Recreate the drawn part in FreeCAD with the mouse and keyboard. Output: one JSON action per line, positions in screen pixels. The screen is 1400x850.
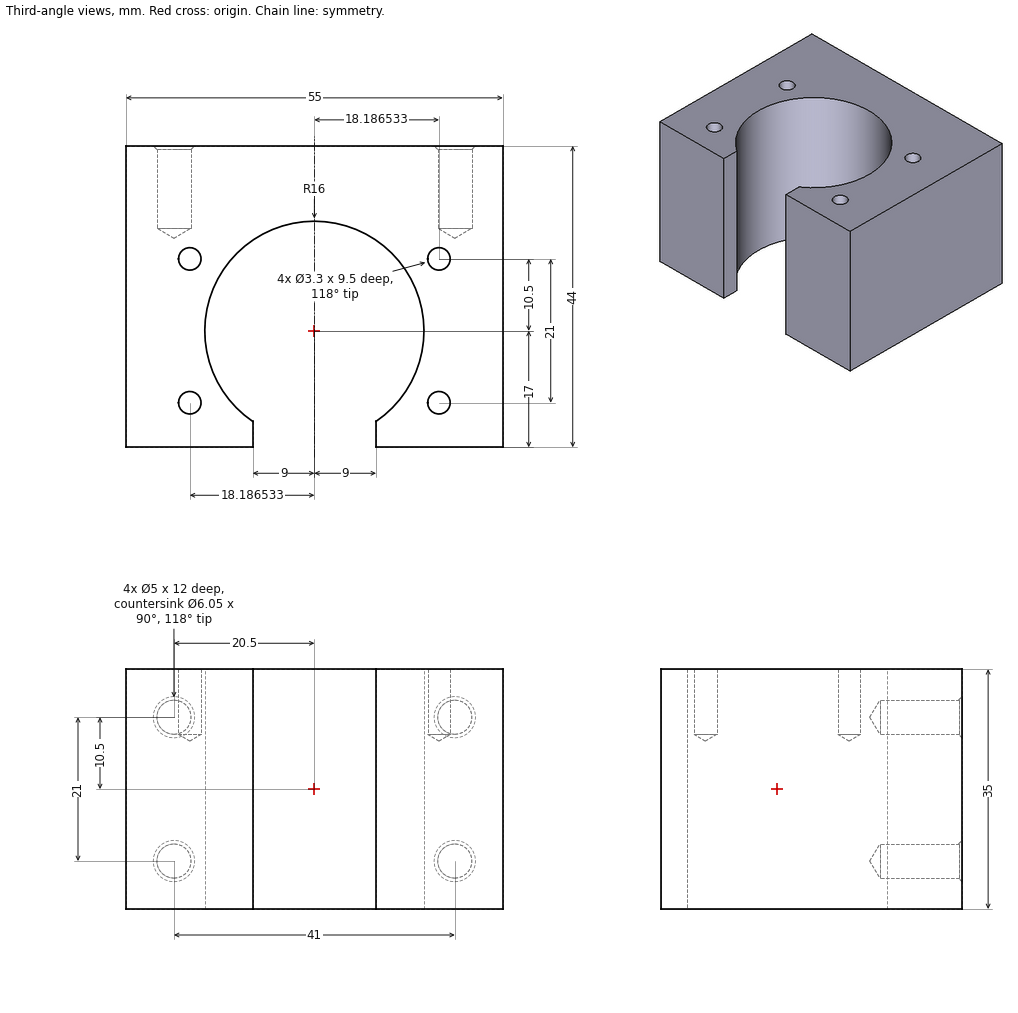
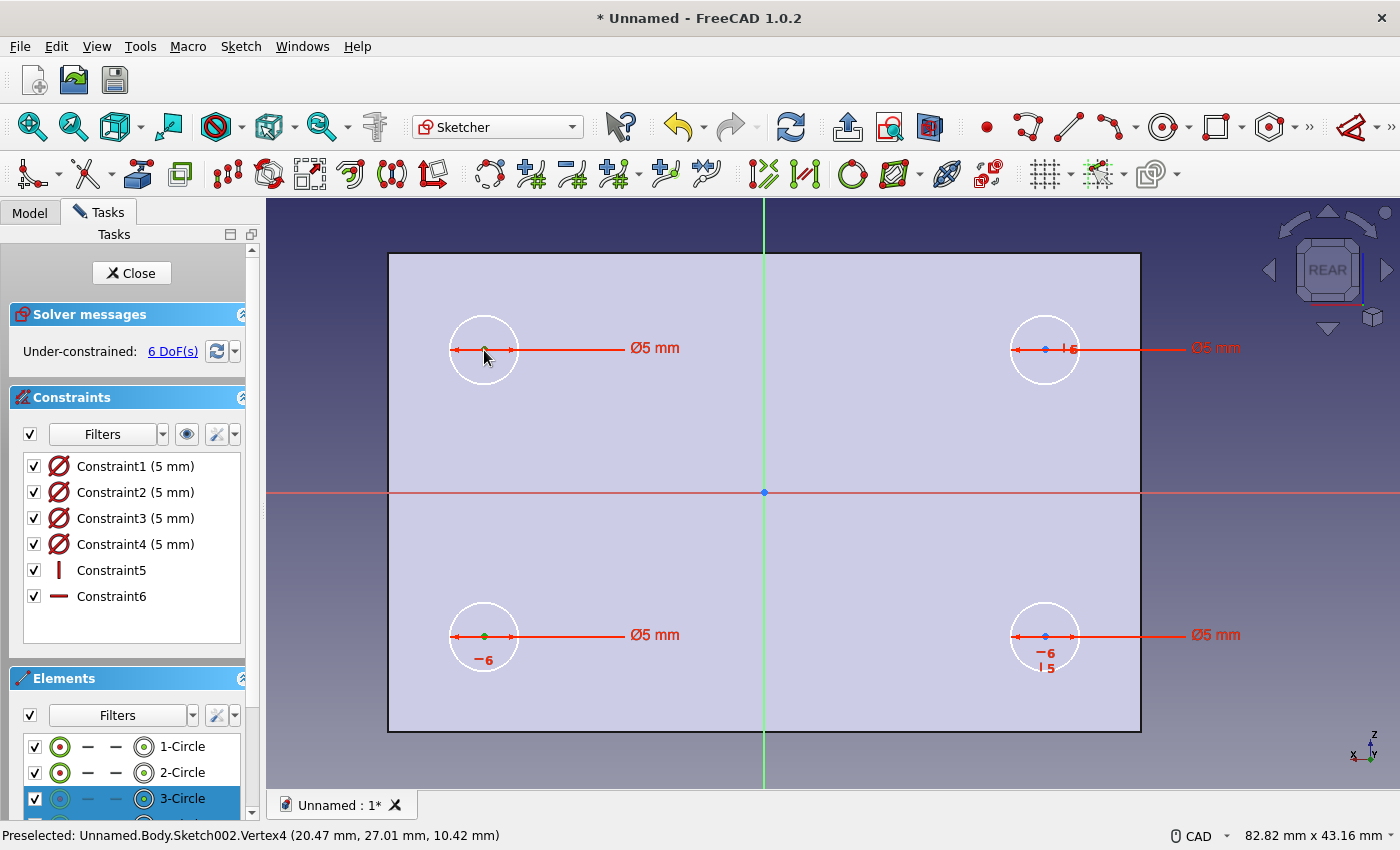
{"action": "key", "text": "v"}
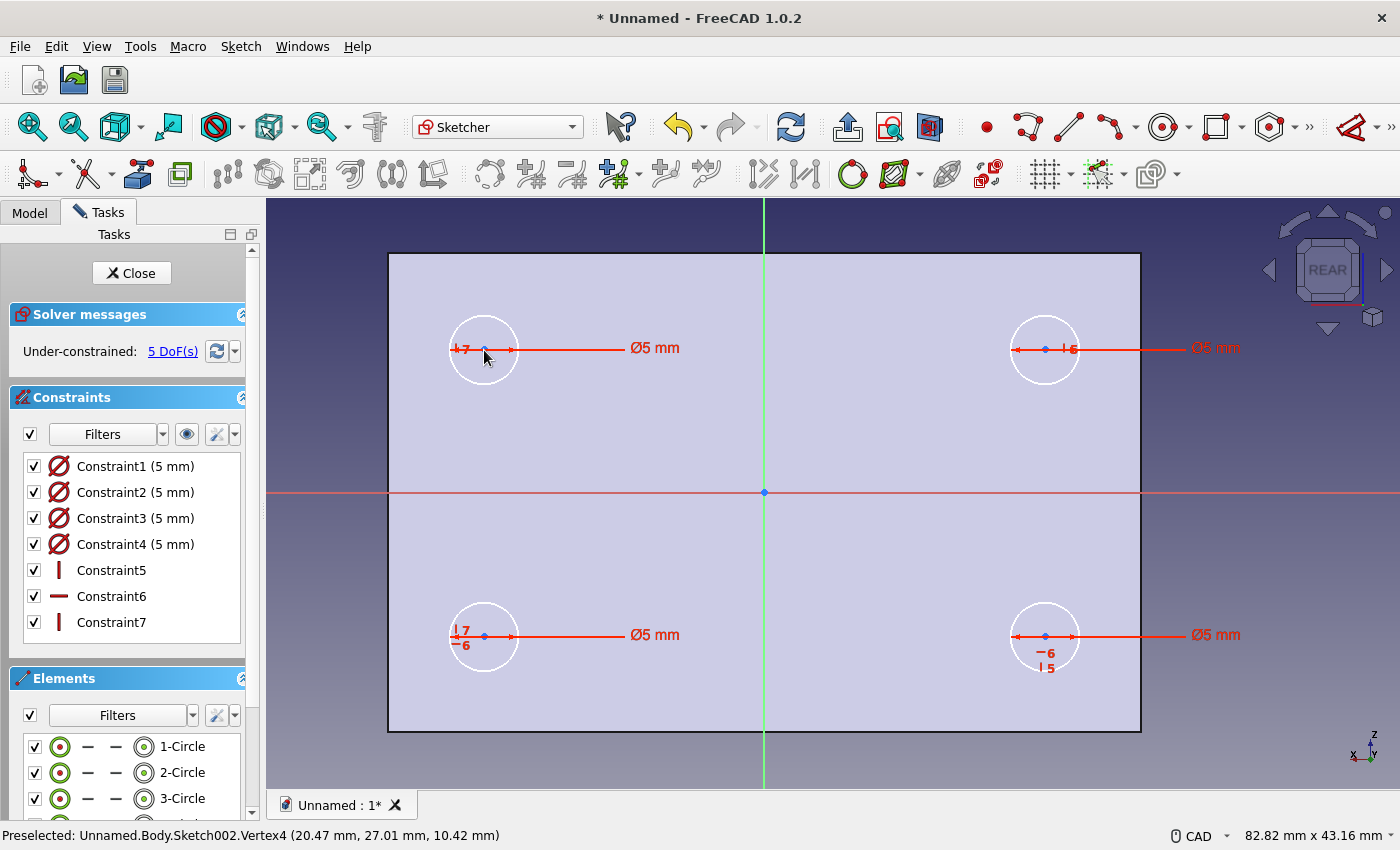
{"action": "left_click", "coordinate": [1045, 350]}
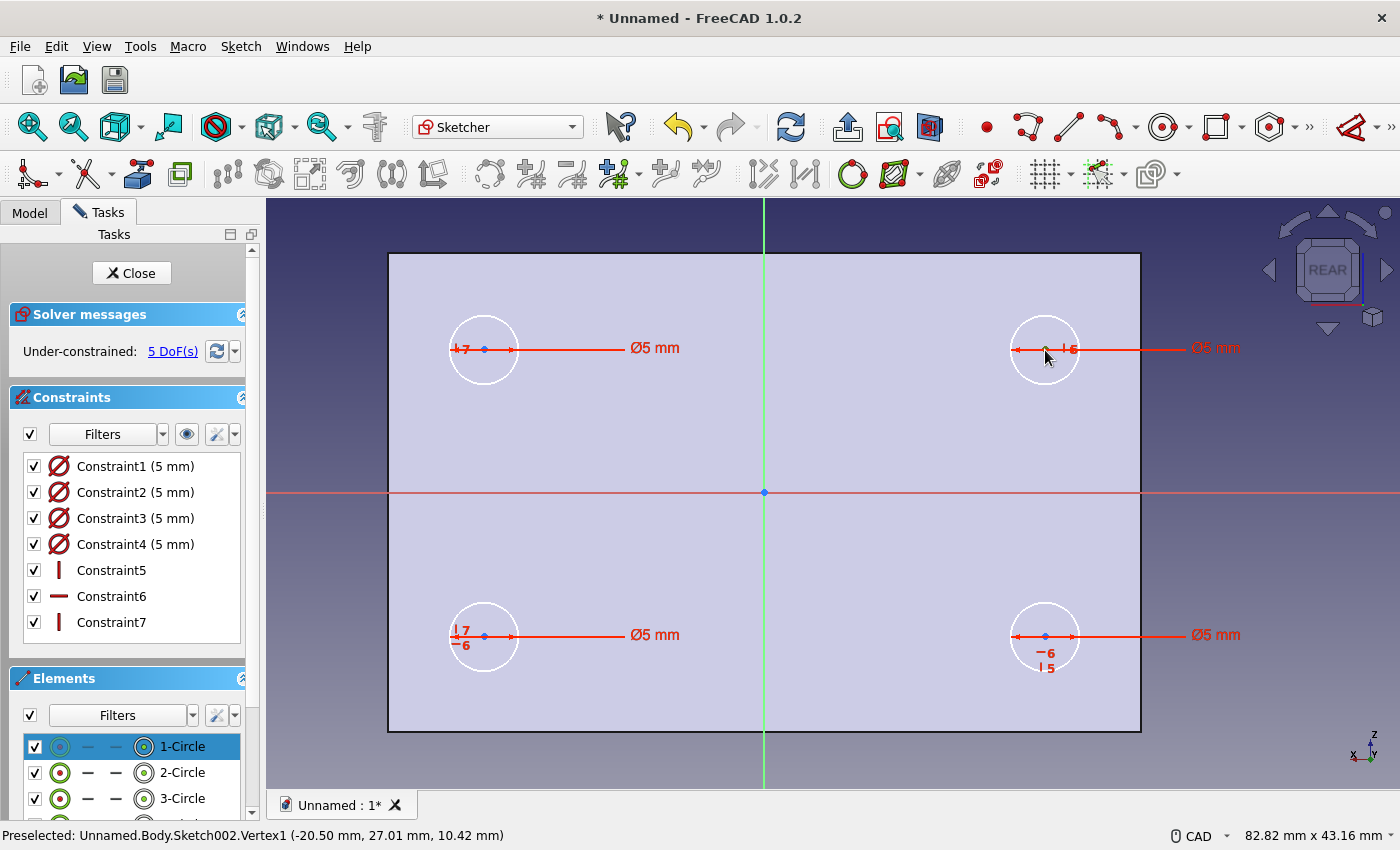
{"action": "left_click", "coordinate": [484, 350]}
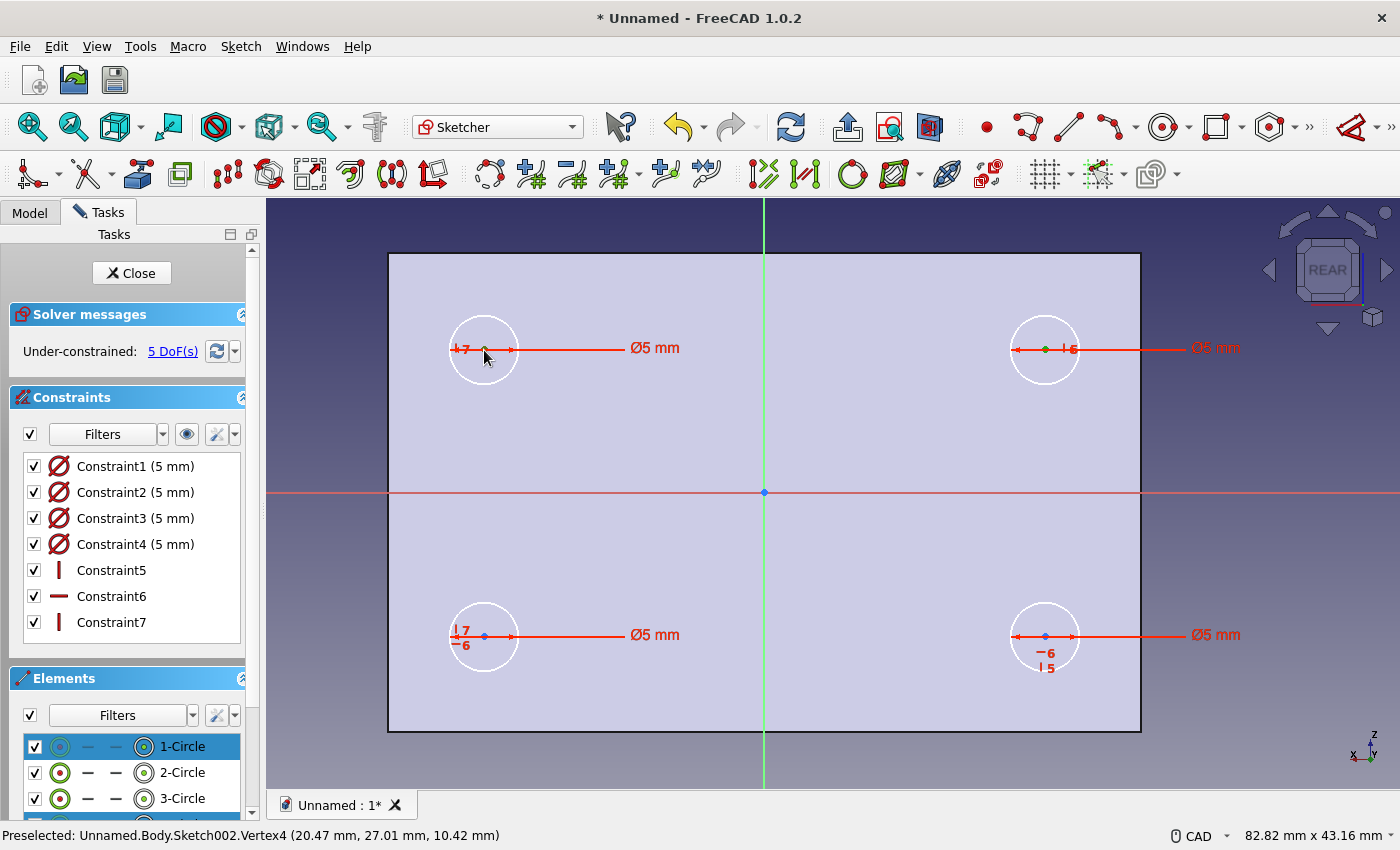
{"action": "key", "text": "h"}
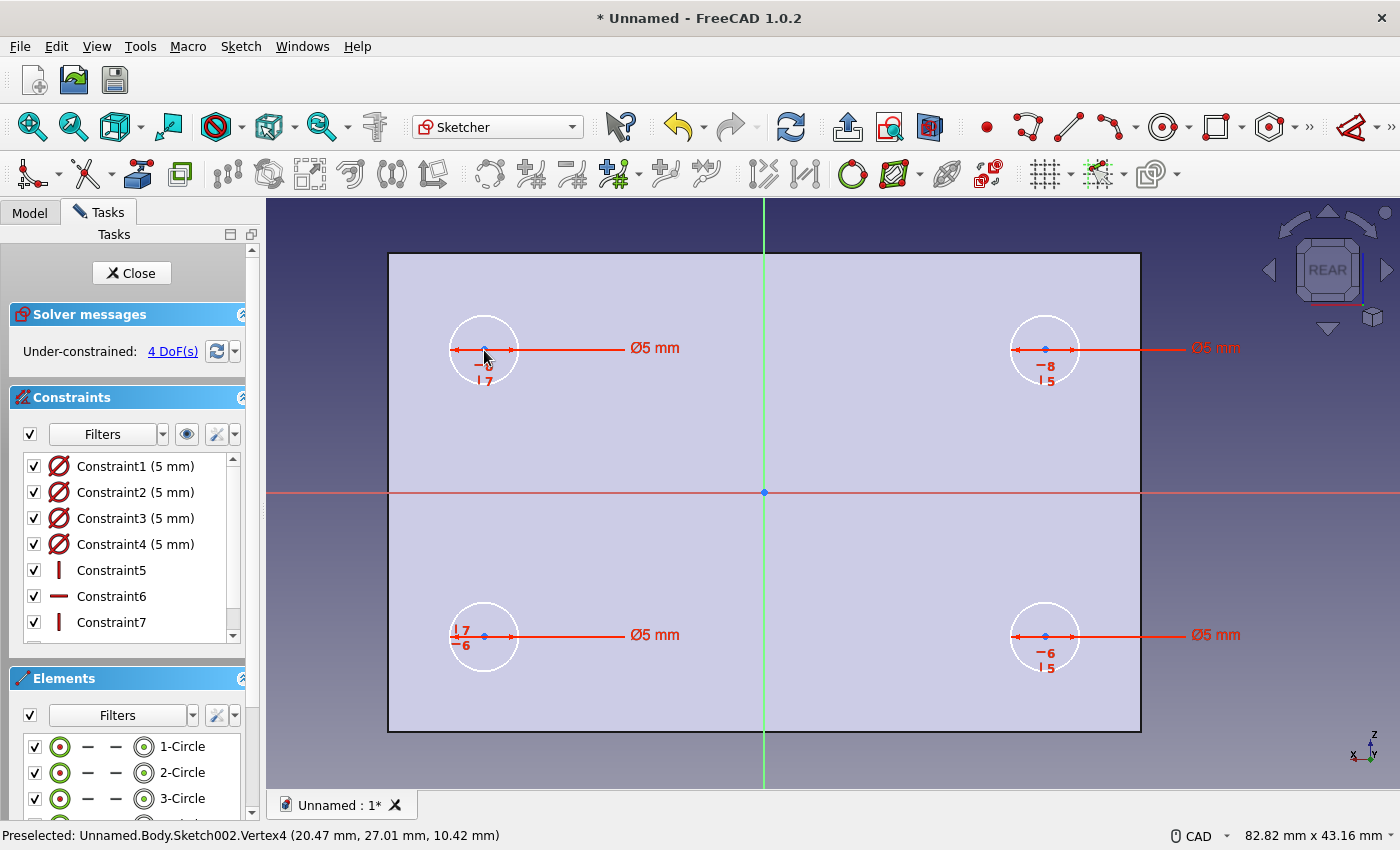
{"action": "left_click", "coordinate": [1350, 128]}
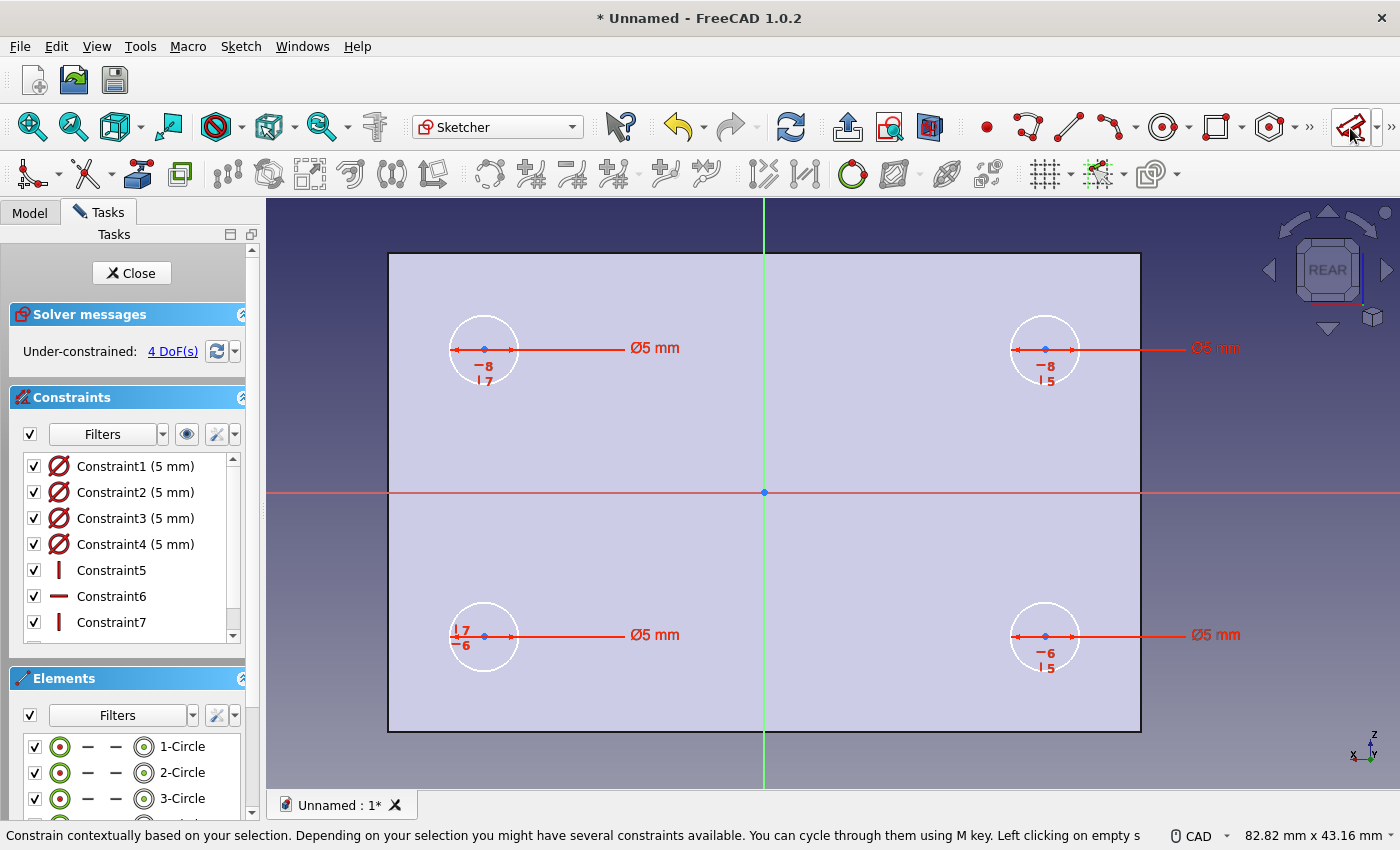
{"action": "left_click", "coordinate": [1045, 350]}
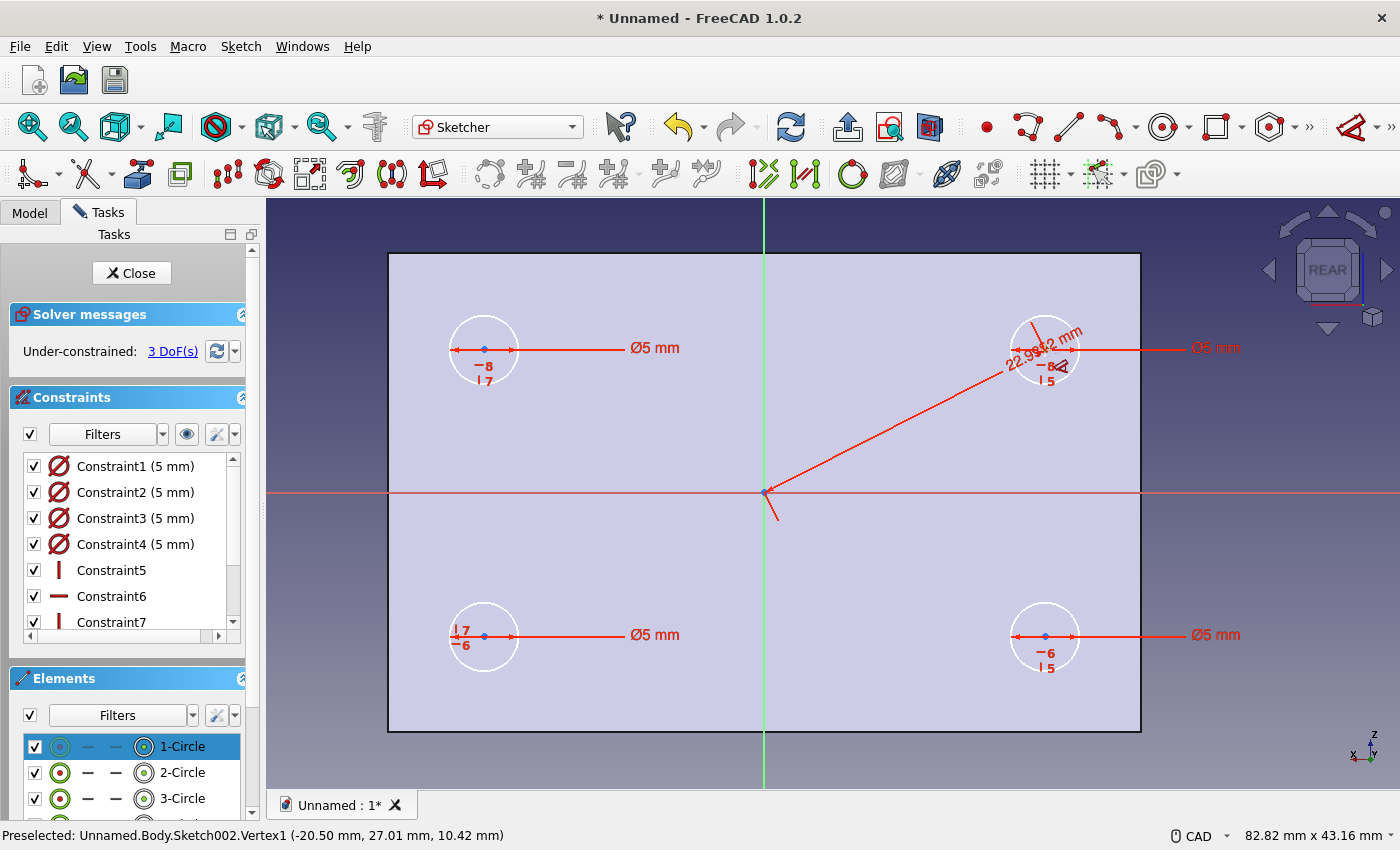
{"action": "left_click", "coordinate": [1045, 637]}
{"action": "left_click", "coordinate": [1079, 427]}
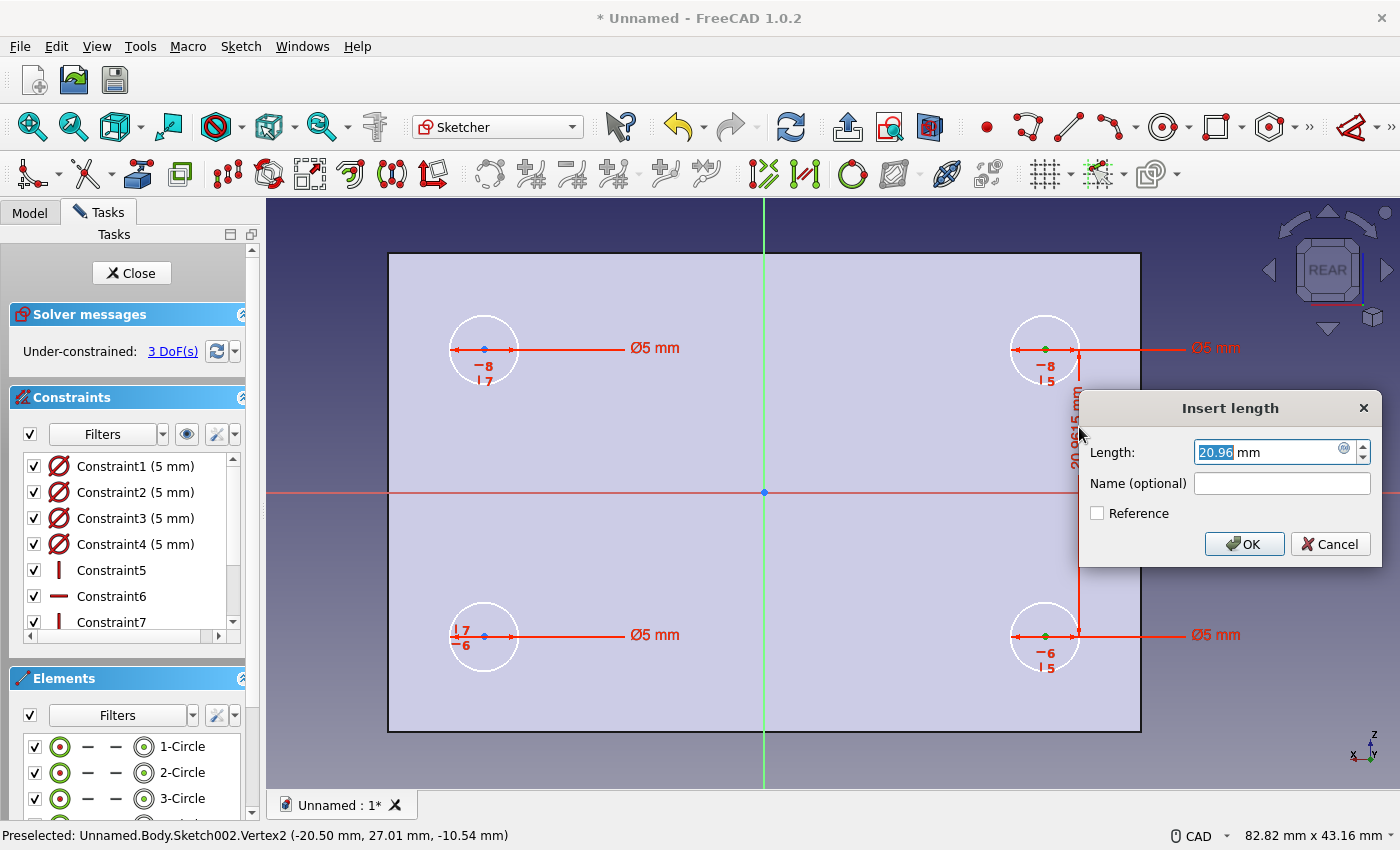
{"action": "type", "text": "21"}
{"action": "key", "text": "Return"}